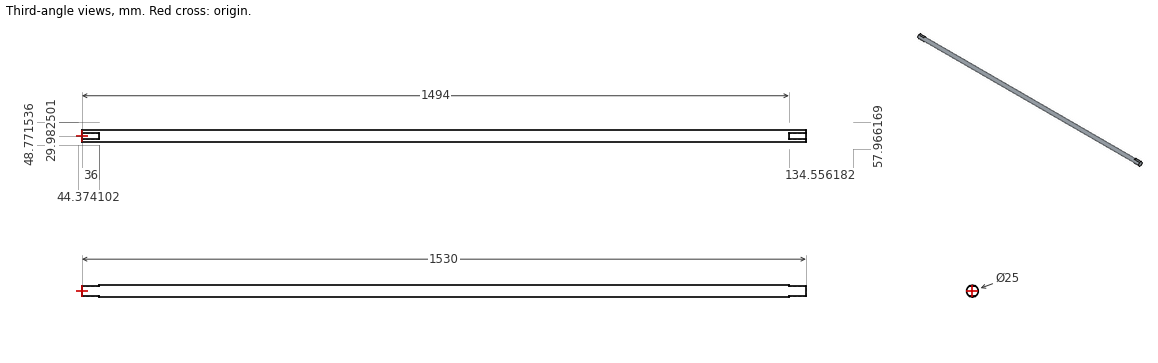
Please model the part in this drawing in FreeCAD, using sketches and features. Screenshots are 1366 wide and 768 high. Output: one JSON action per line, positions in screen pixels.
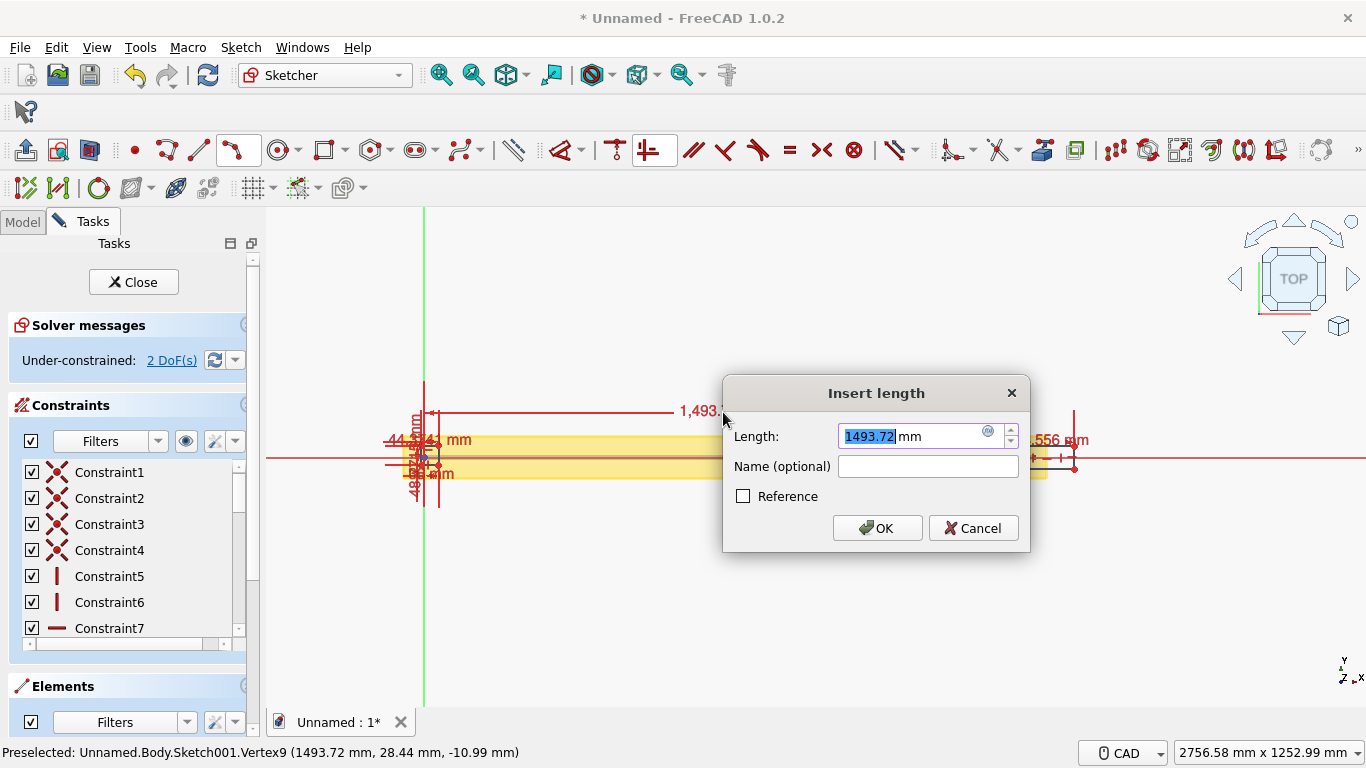
{"action": "type", "text": "1494"}
{"action": "key", "text": "Return"}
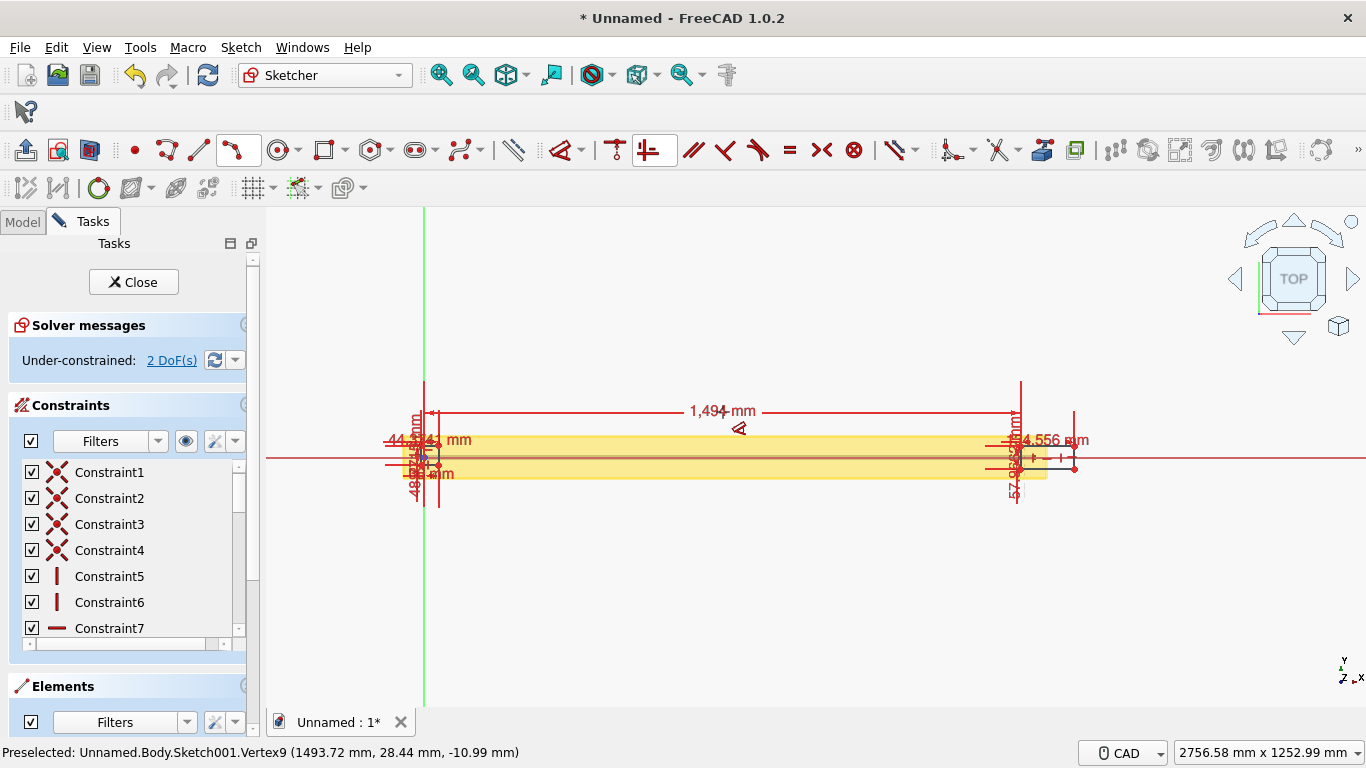
{"action": "scroll", "coordinate": [421, 446], "scroll_direction": "up", "scroll_amount": 6}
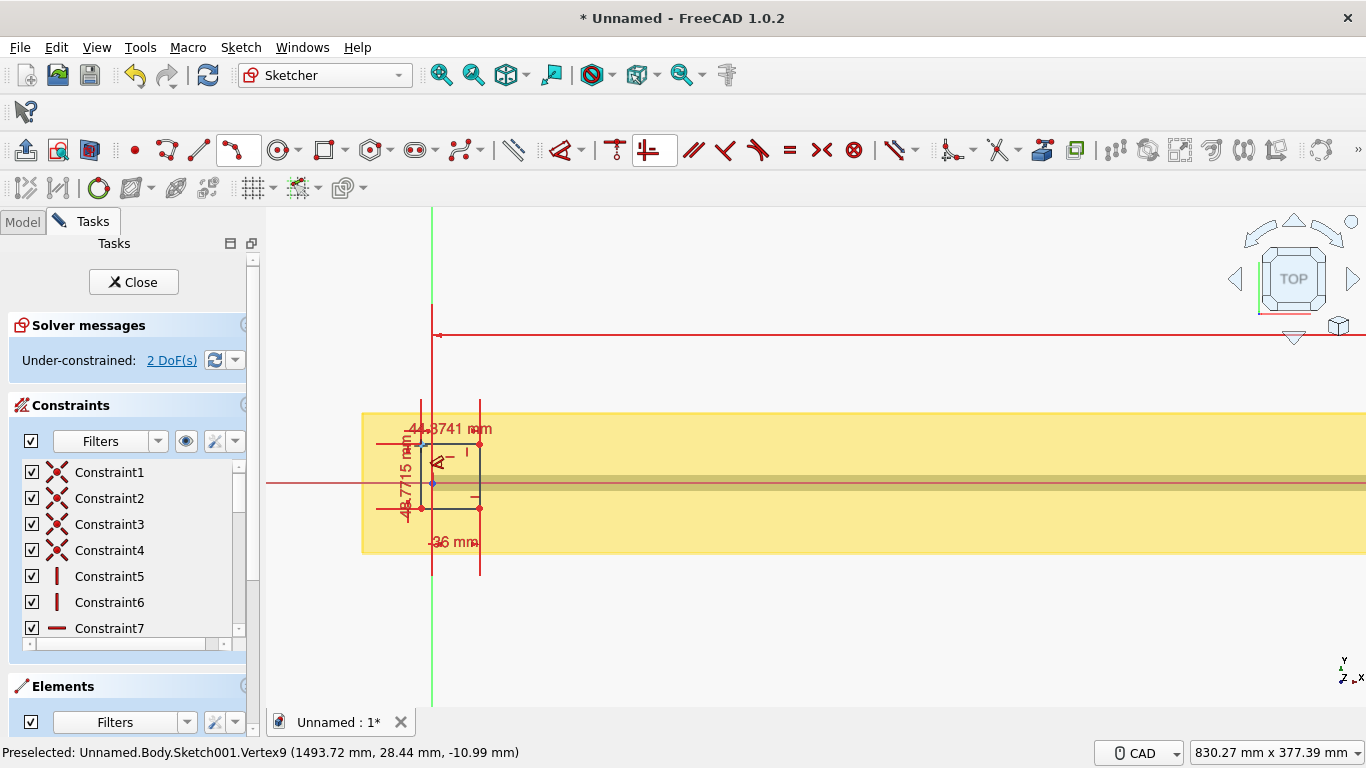
{"action": "left_click", "coordinate": [421, 444]}
{"action": "left_click", "coordinate": [387, 464]}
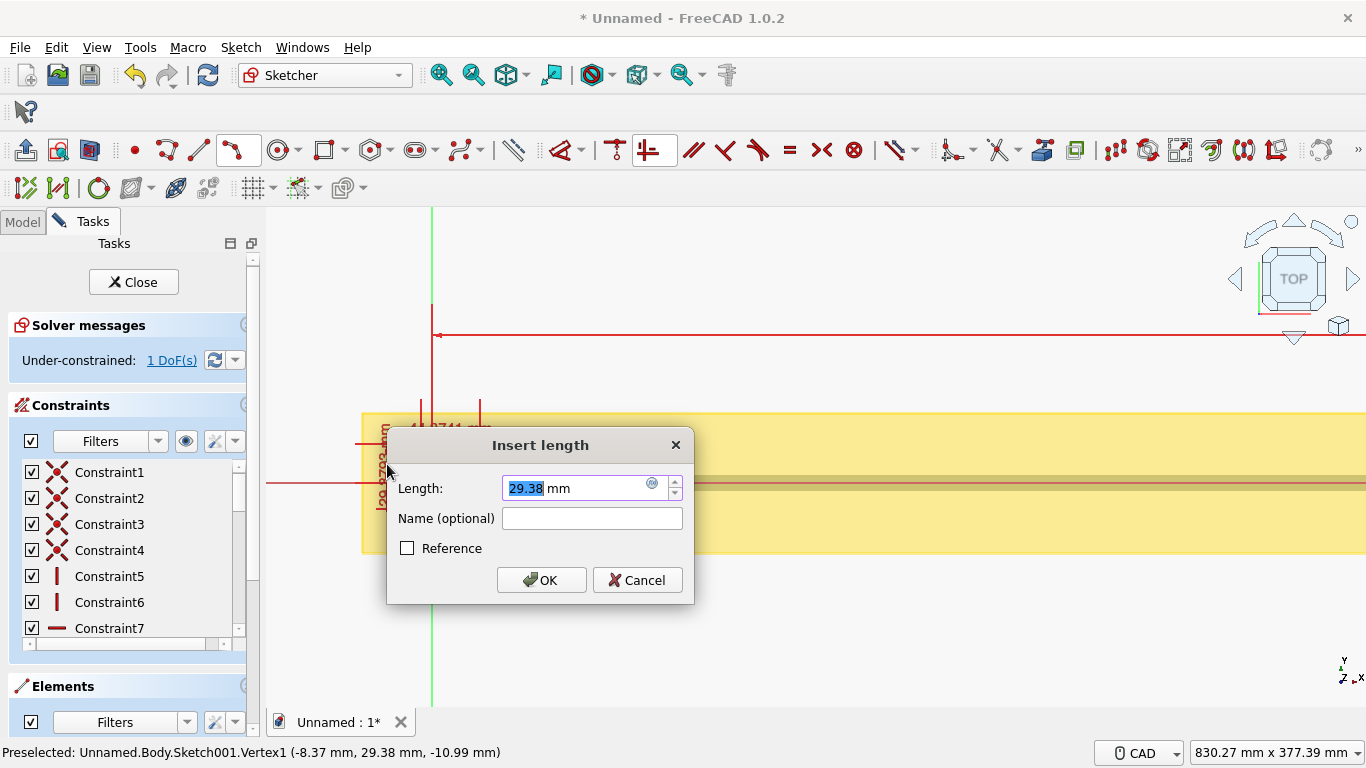
{"action": "type", "text": "29.982501"}
{"action": "key", "text": "Return"}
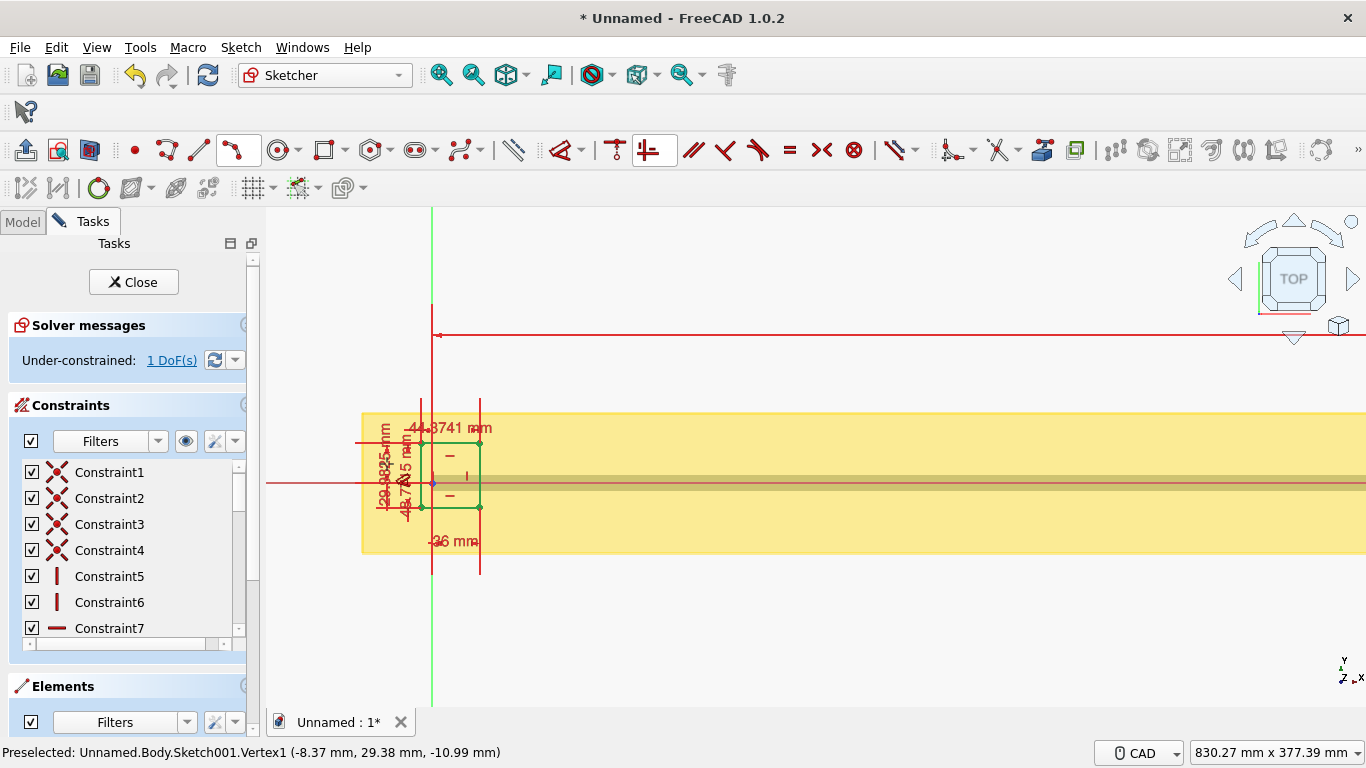
{"action": "scroll", "coordinate": [421, 446], "scroll_direction": "down", "scroll_amount": 6}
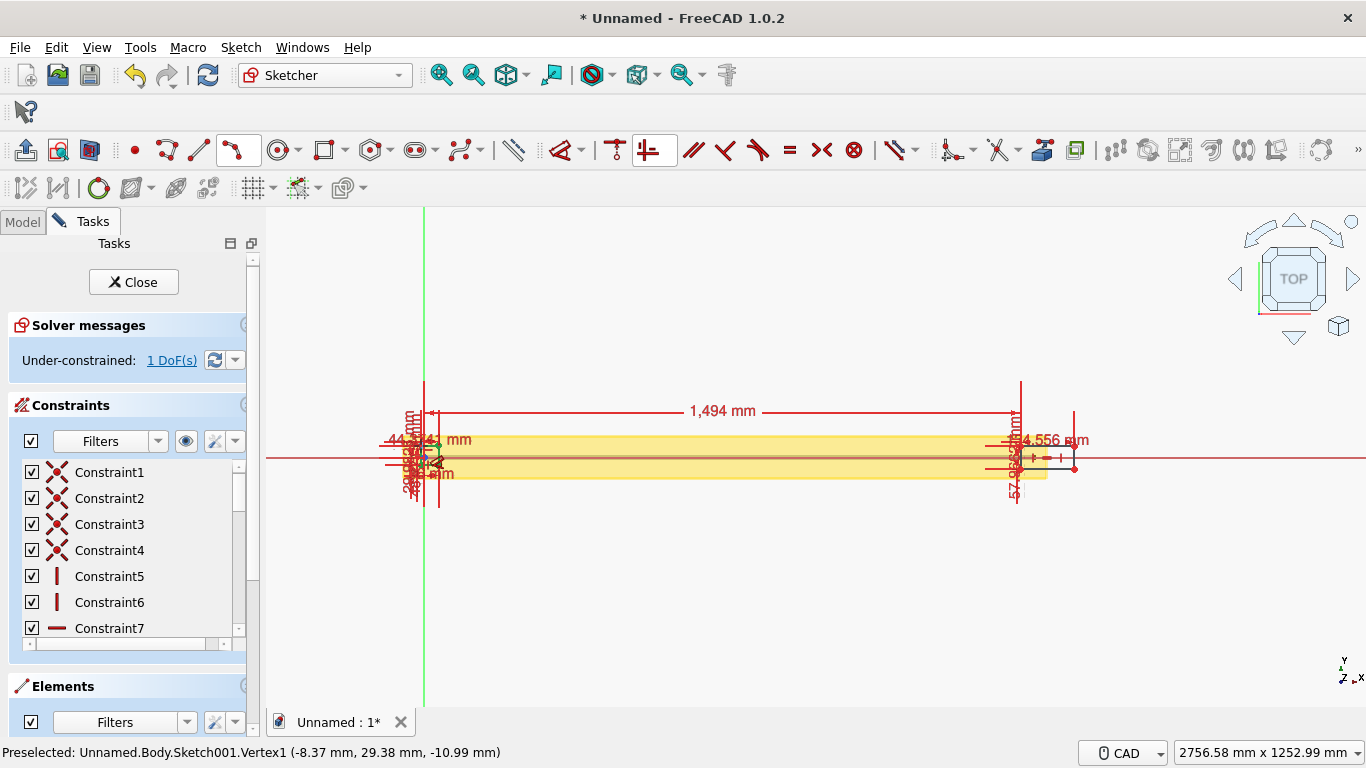
{"action": "scroll", "coordinate": [1021, 446], "scroll_direction": "up", "scroll_amount": 6}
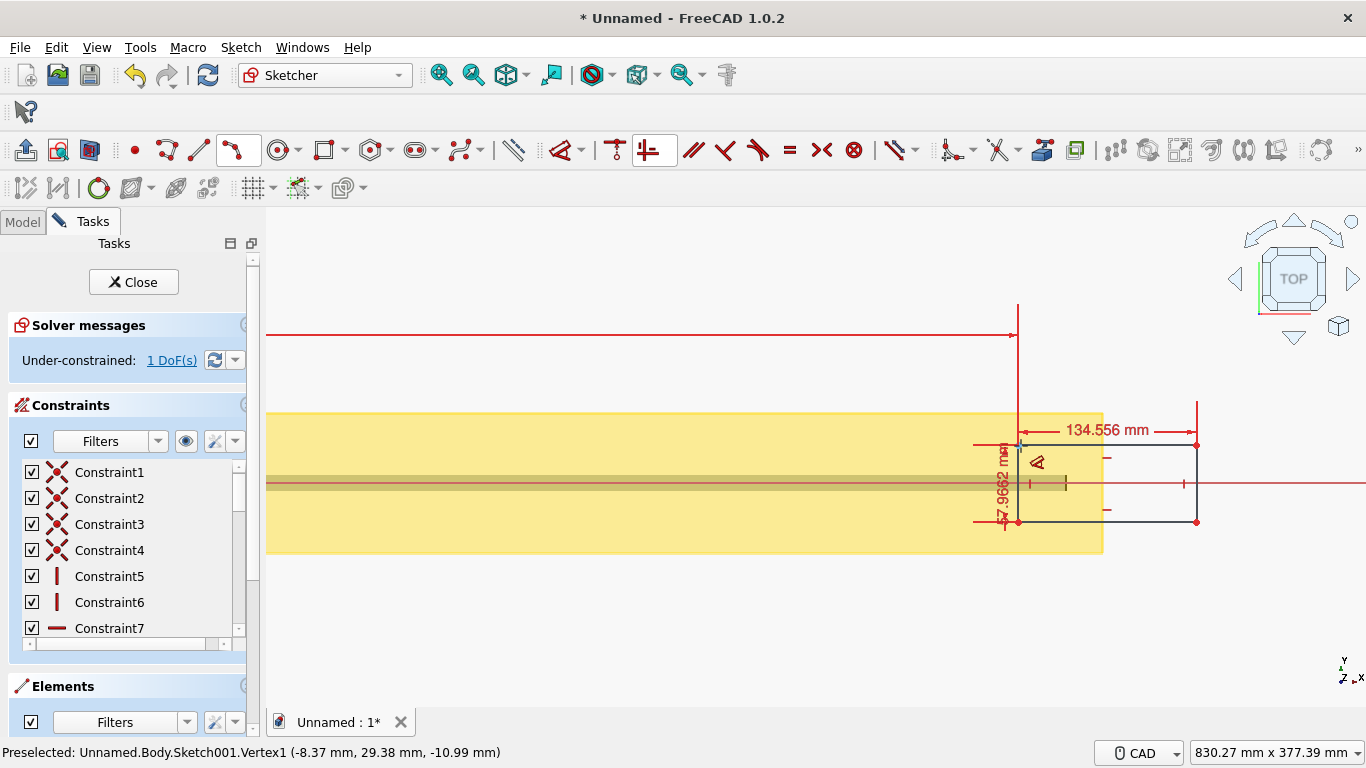
{"action": "left_click", "coordinate": [1018, 445]}
{"action": "left_click", "coordinate": [1052, 464]}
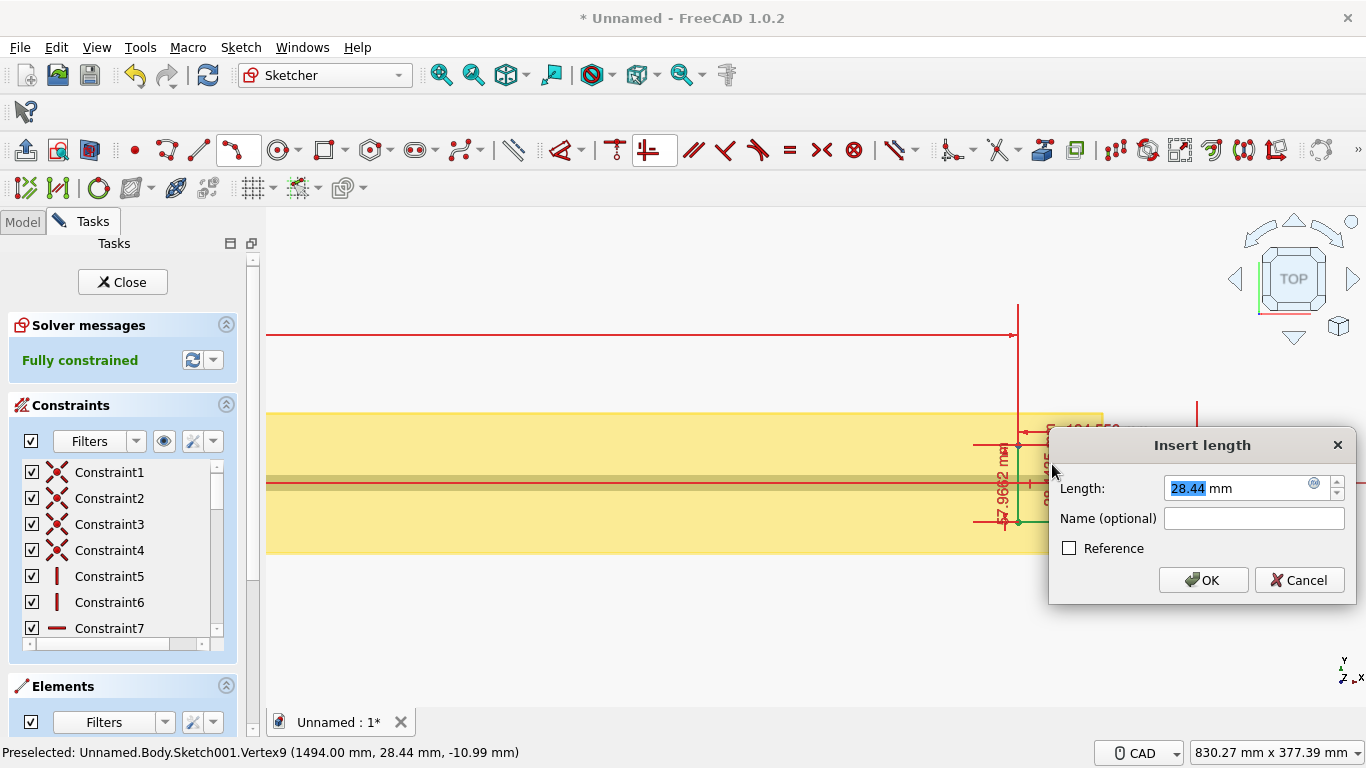
{"action": "type", "text": "29.982501"}
{"action": "key", "text": "Return"}
{"action": "key", "text": "Escape"}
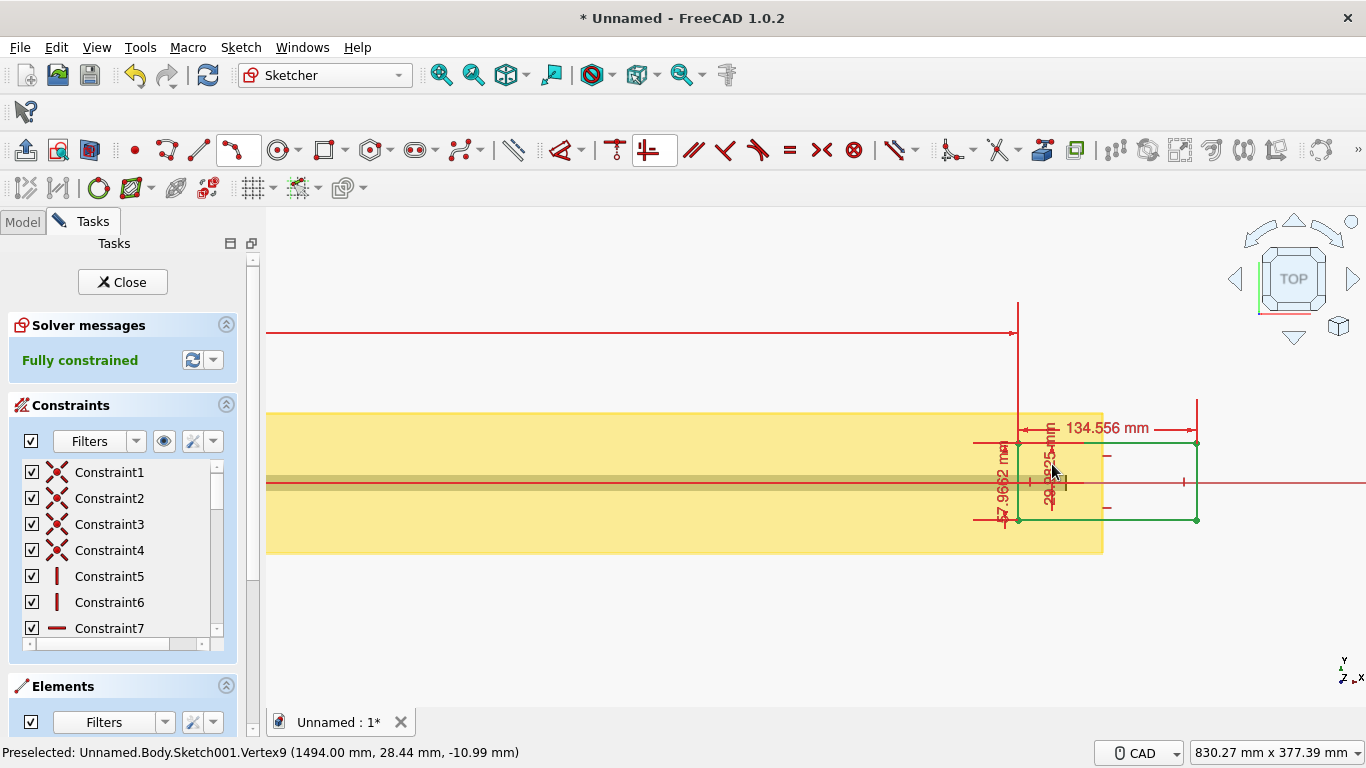
{"action": "left_click", "coordinate": [123, 282]}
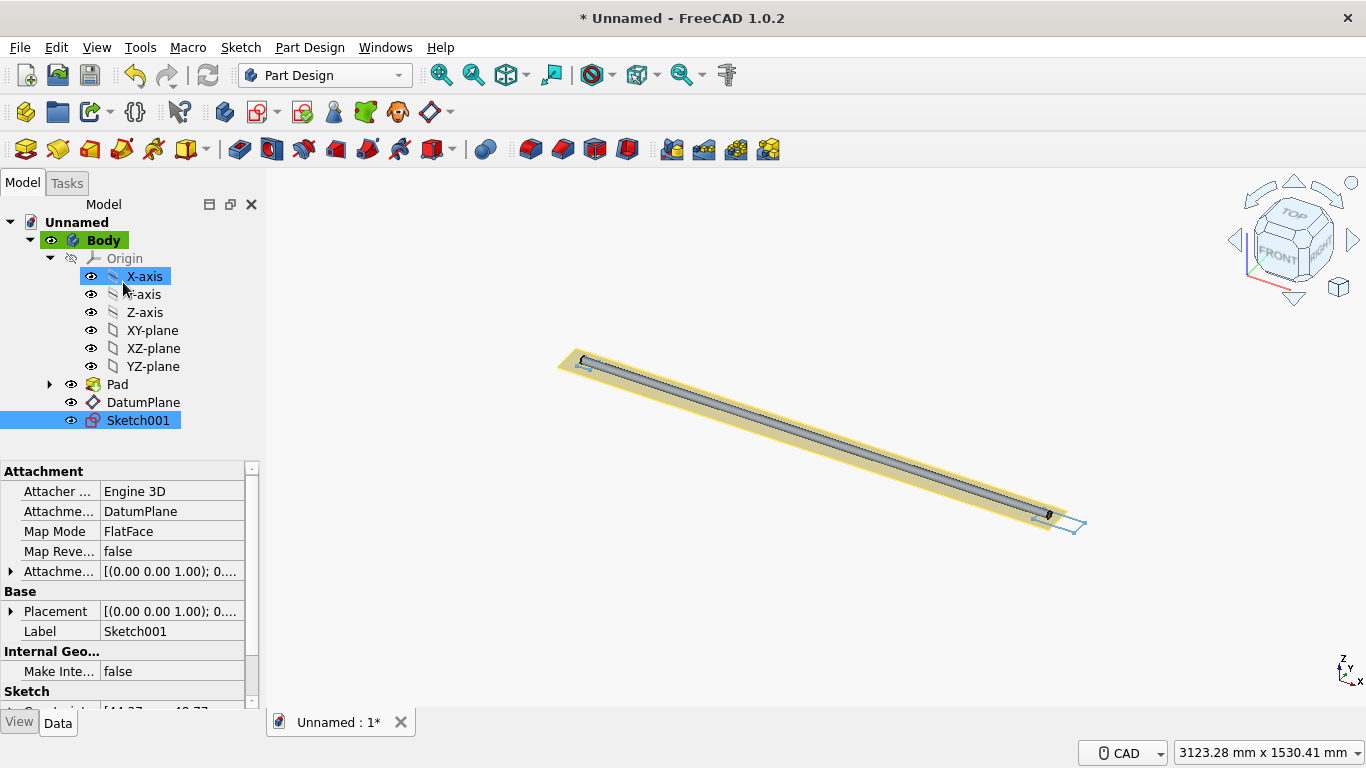
{"action": "left_click", "coordinate": [240, 150]}